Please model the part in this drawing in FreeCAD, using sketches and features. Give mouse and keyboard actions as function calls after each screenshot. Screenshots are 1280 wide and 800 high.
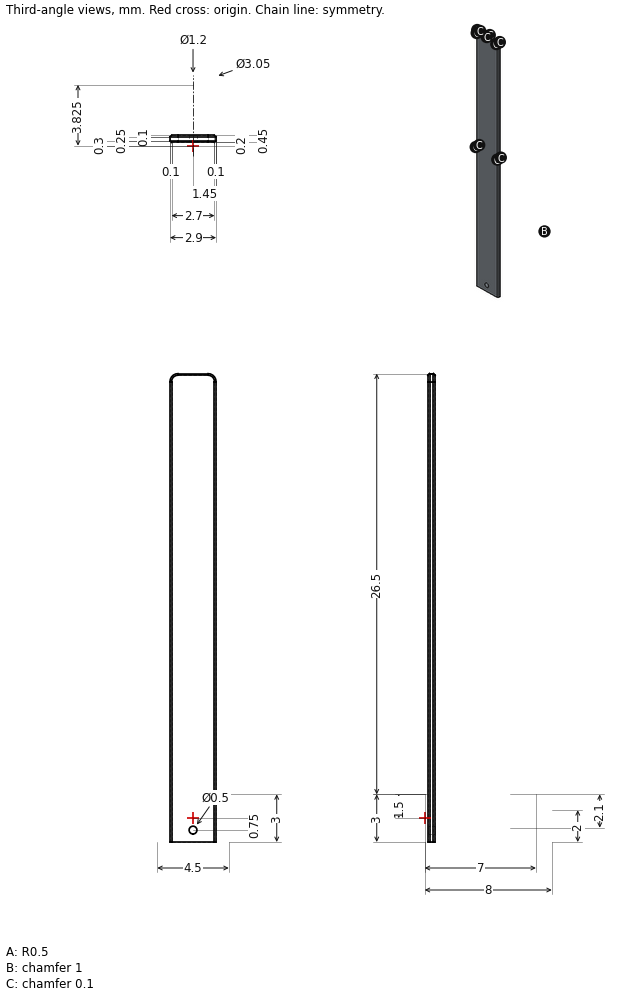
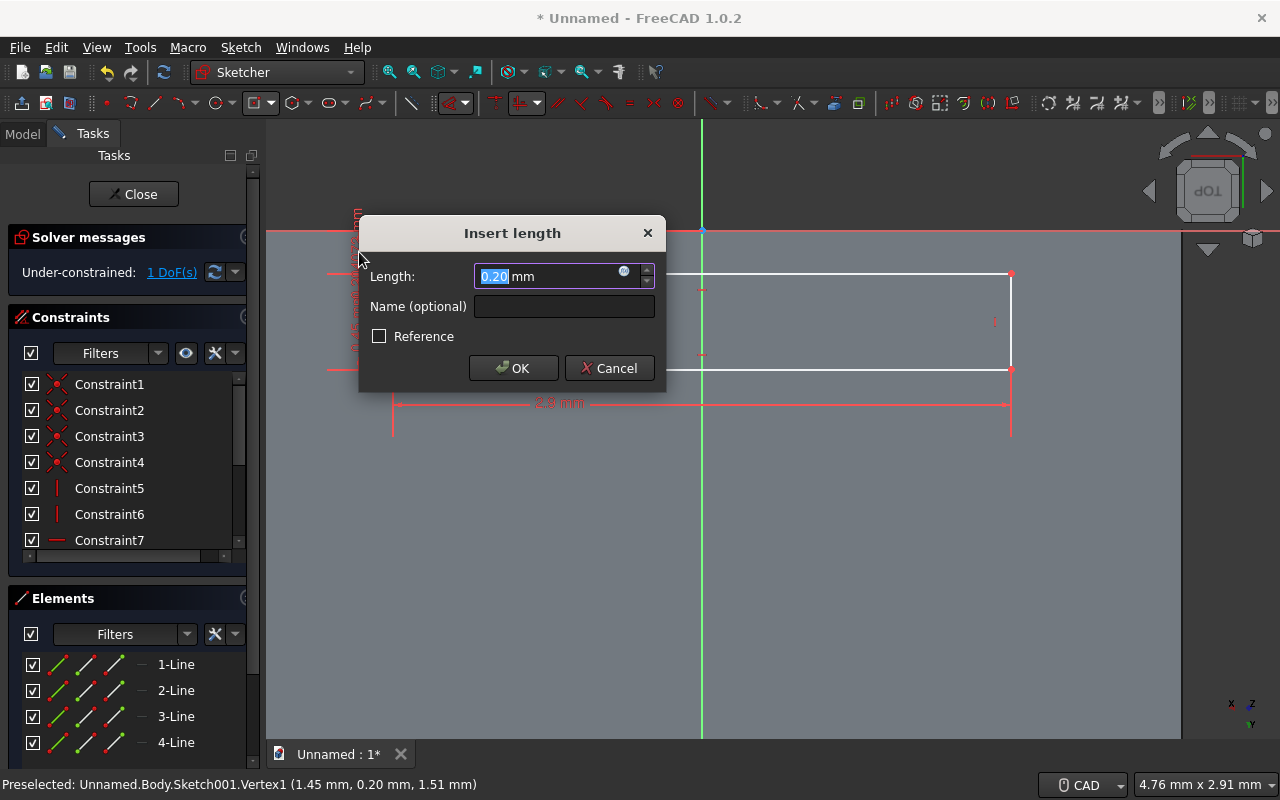
text(0.2)
key(Return)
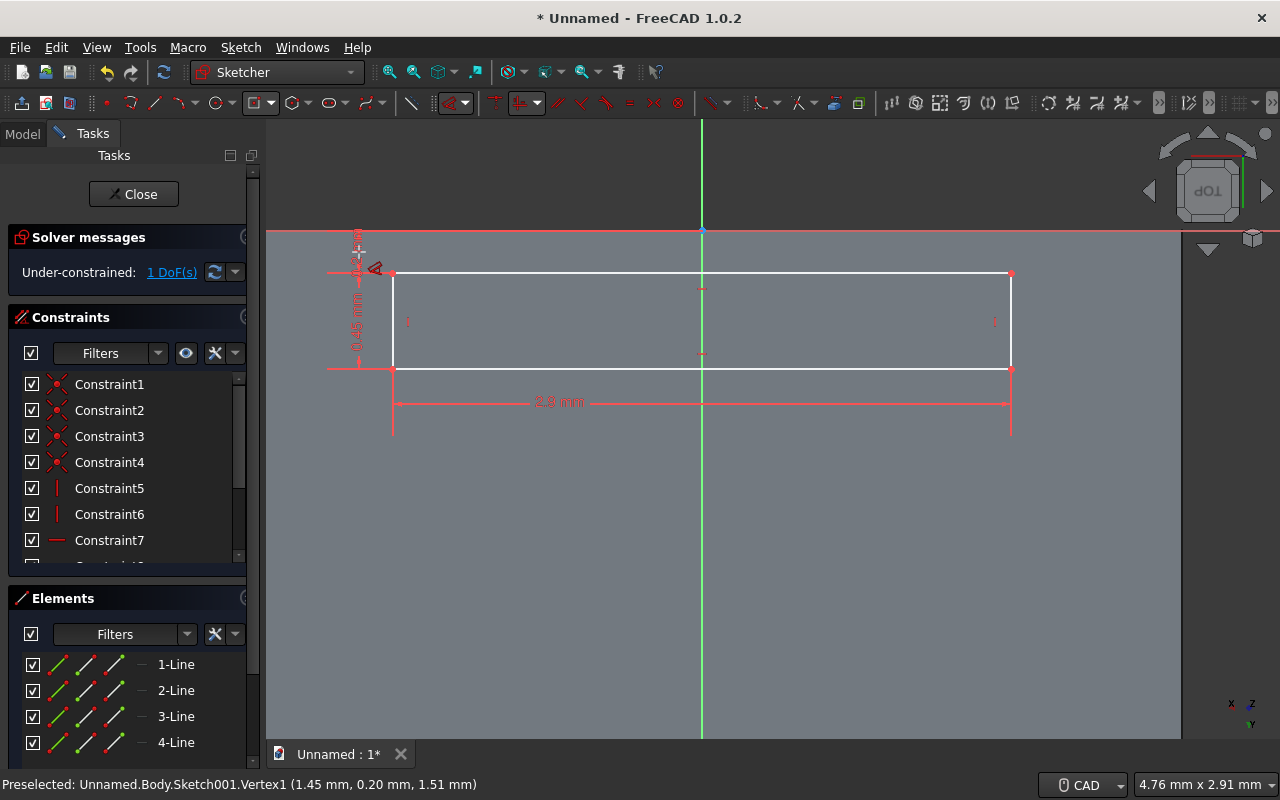
click(393, 273)
click(548, 196)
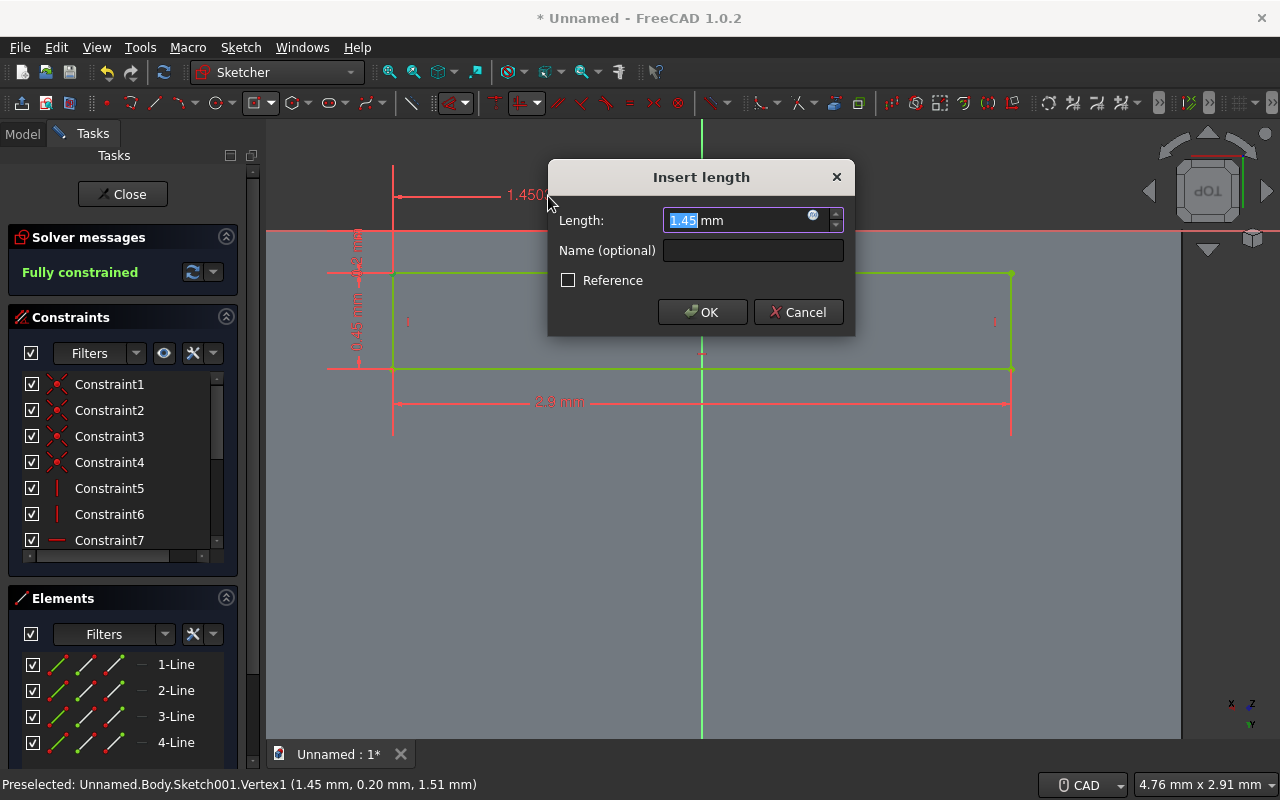
text(1.45)
key(Return)
key(Escape)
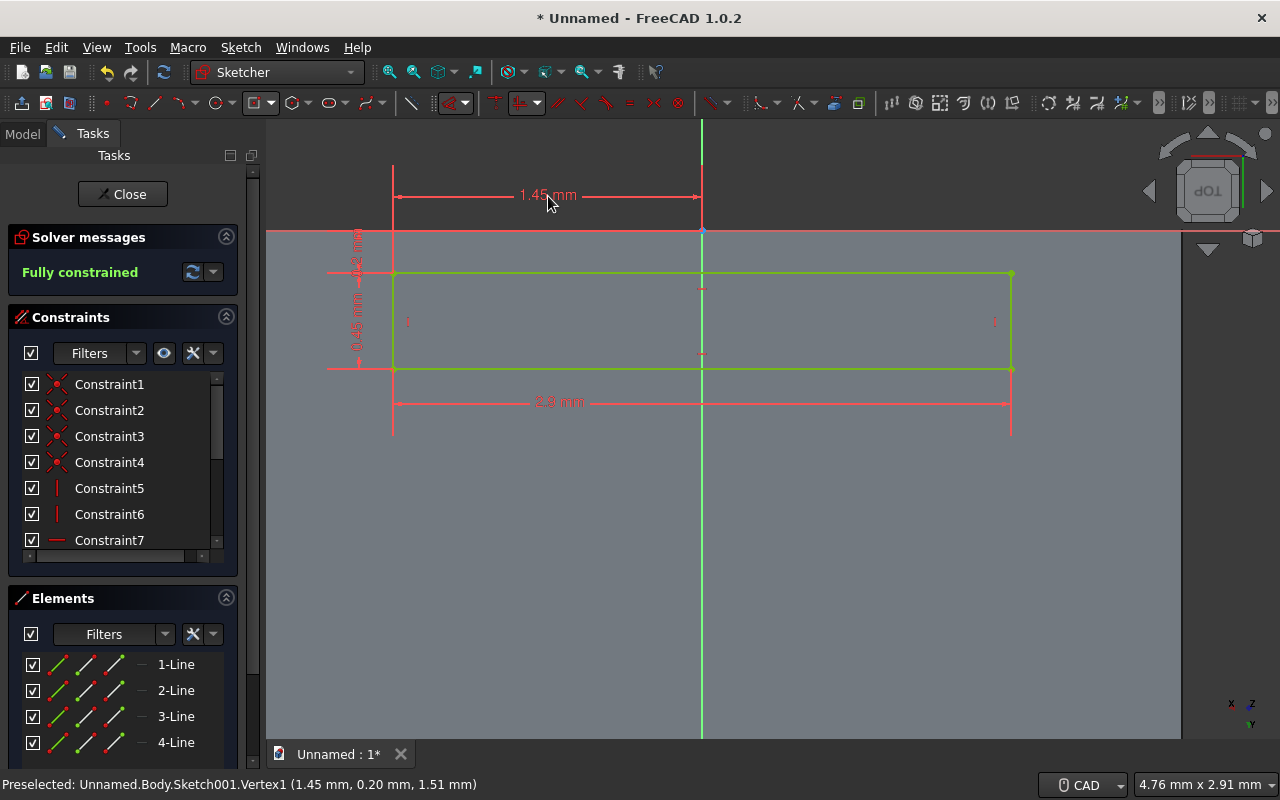
click(123, 194)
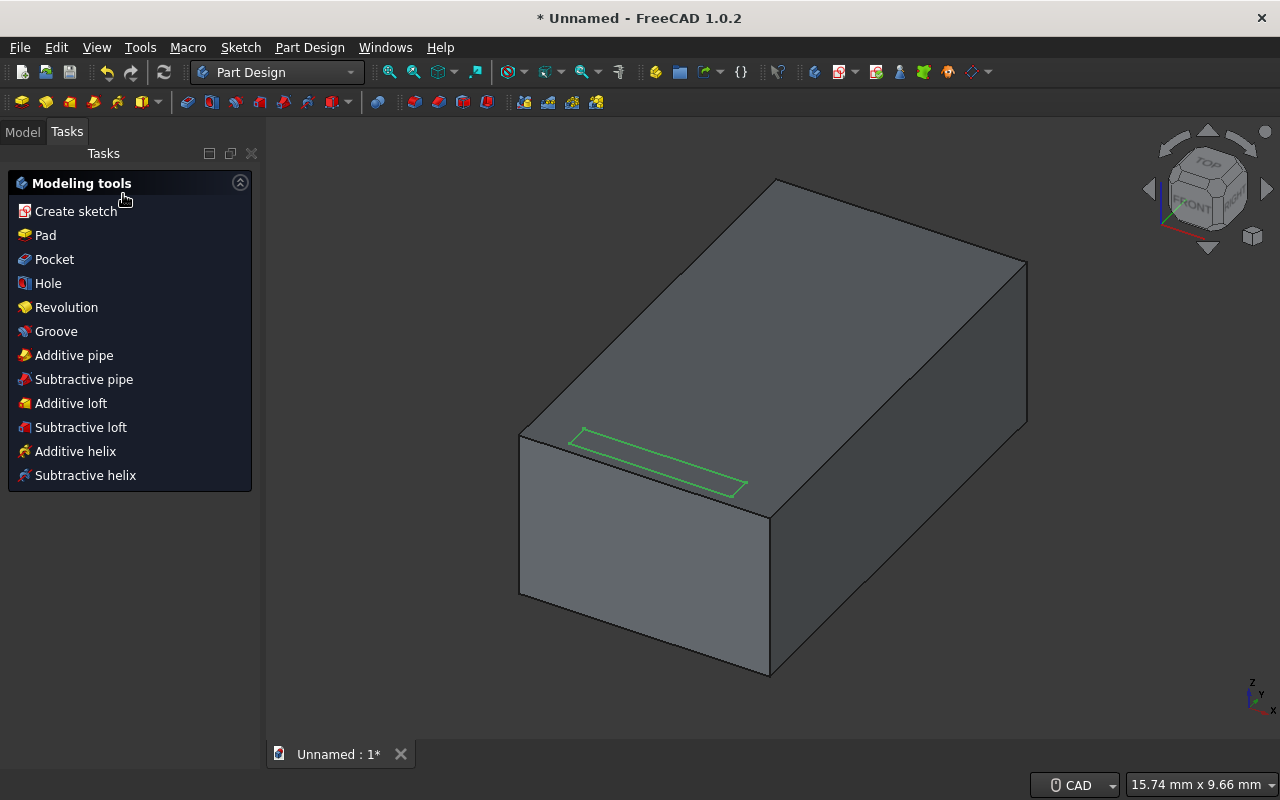
click(22, 102)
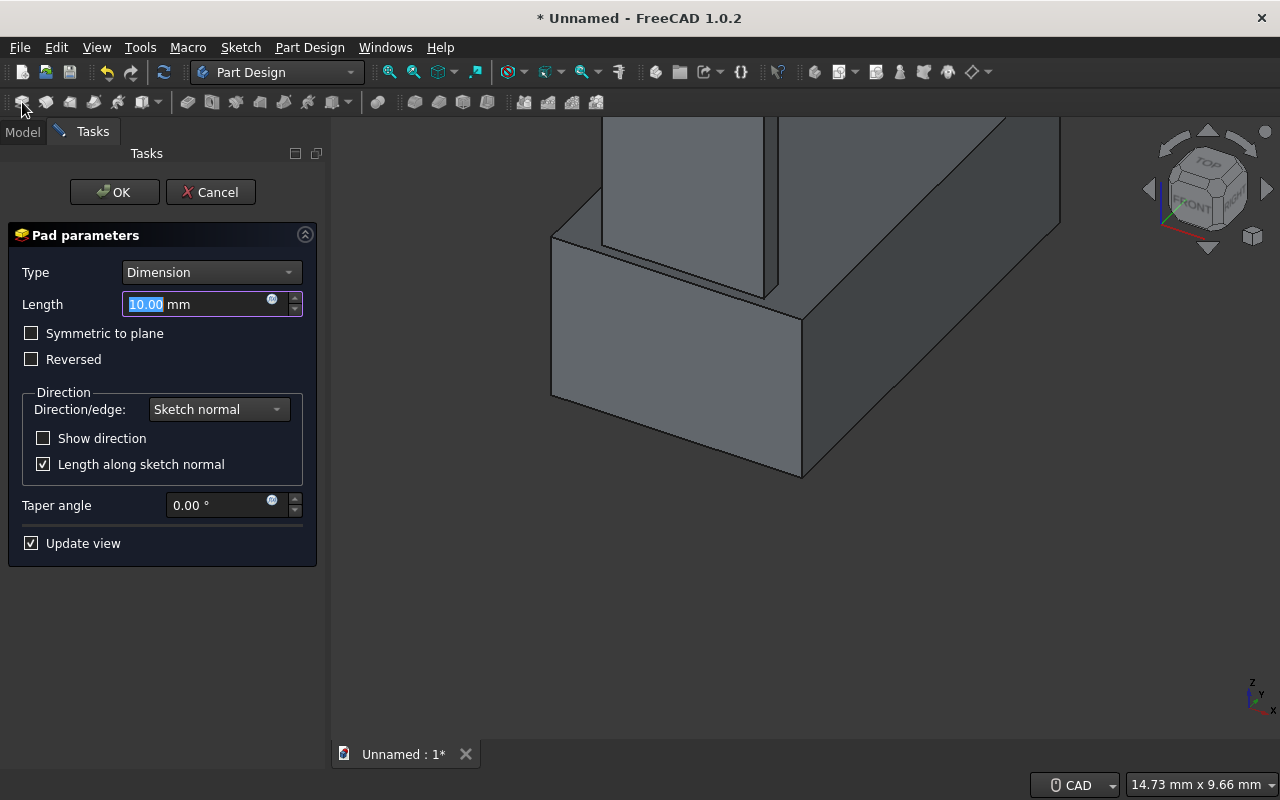
text(26.5)
key(Tab)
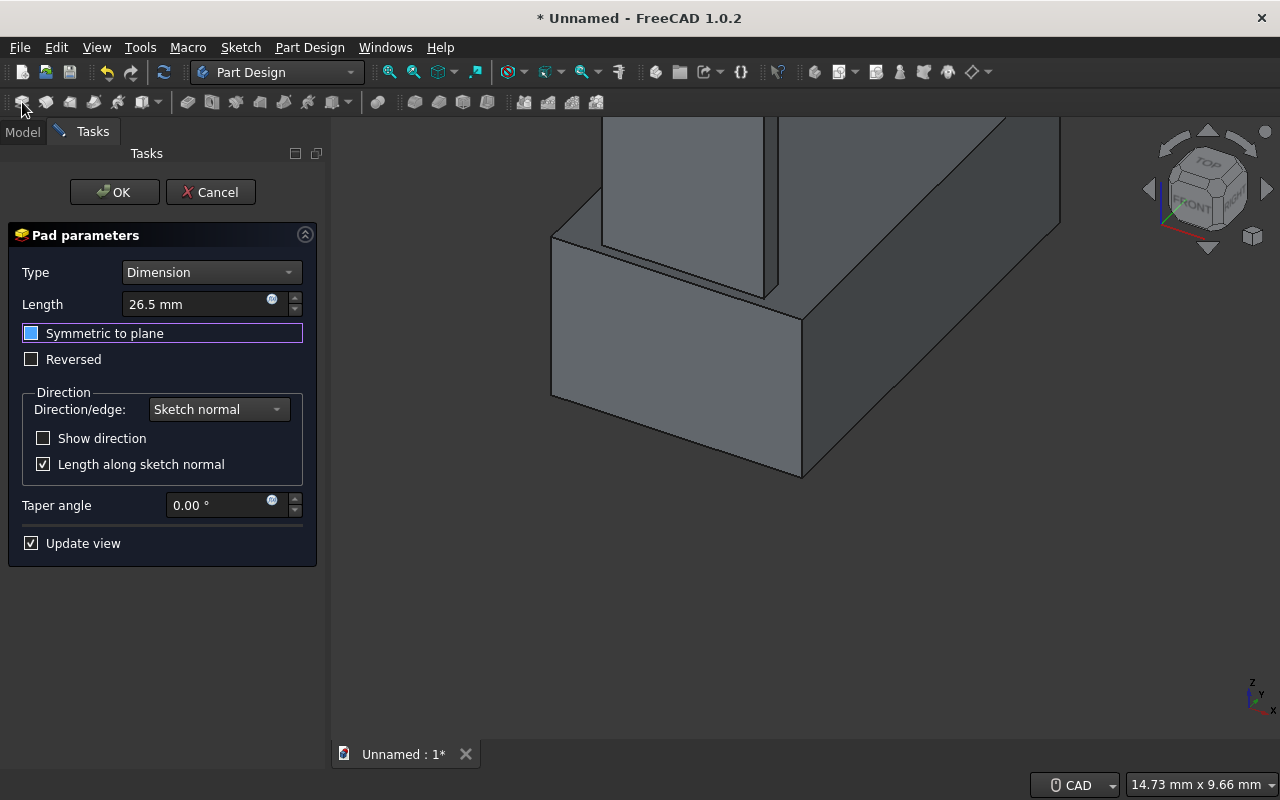
click(115, 192)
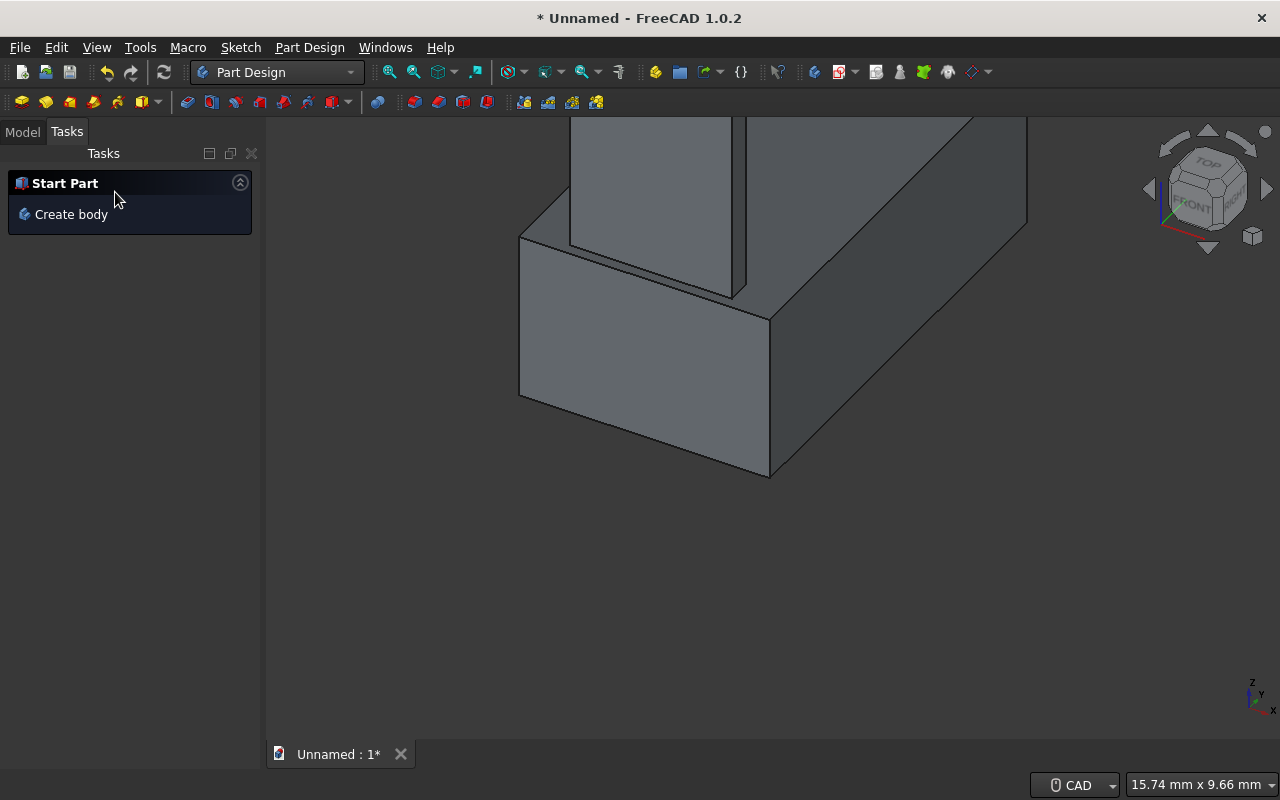
key(v)
key(f)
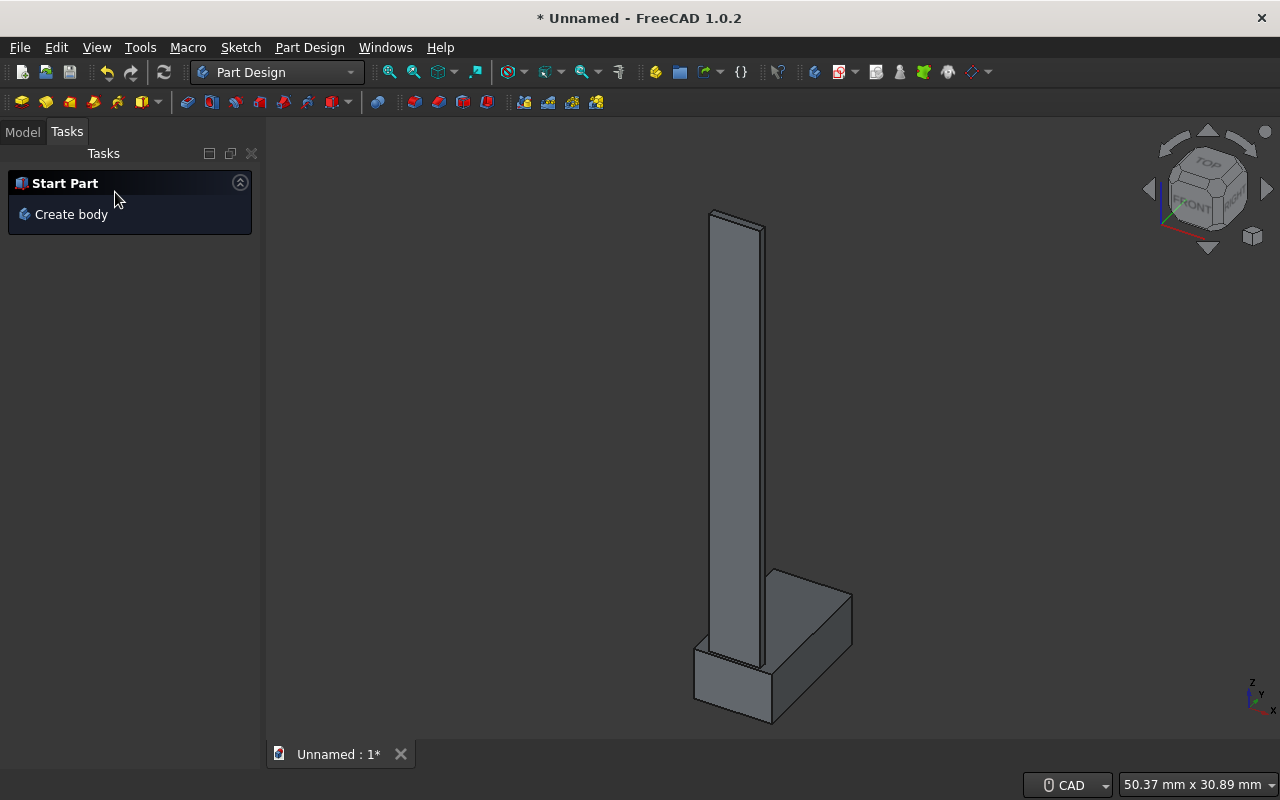
scroll(762, 228, up, 8)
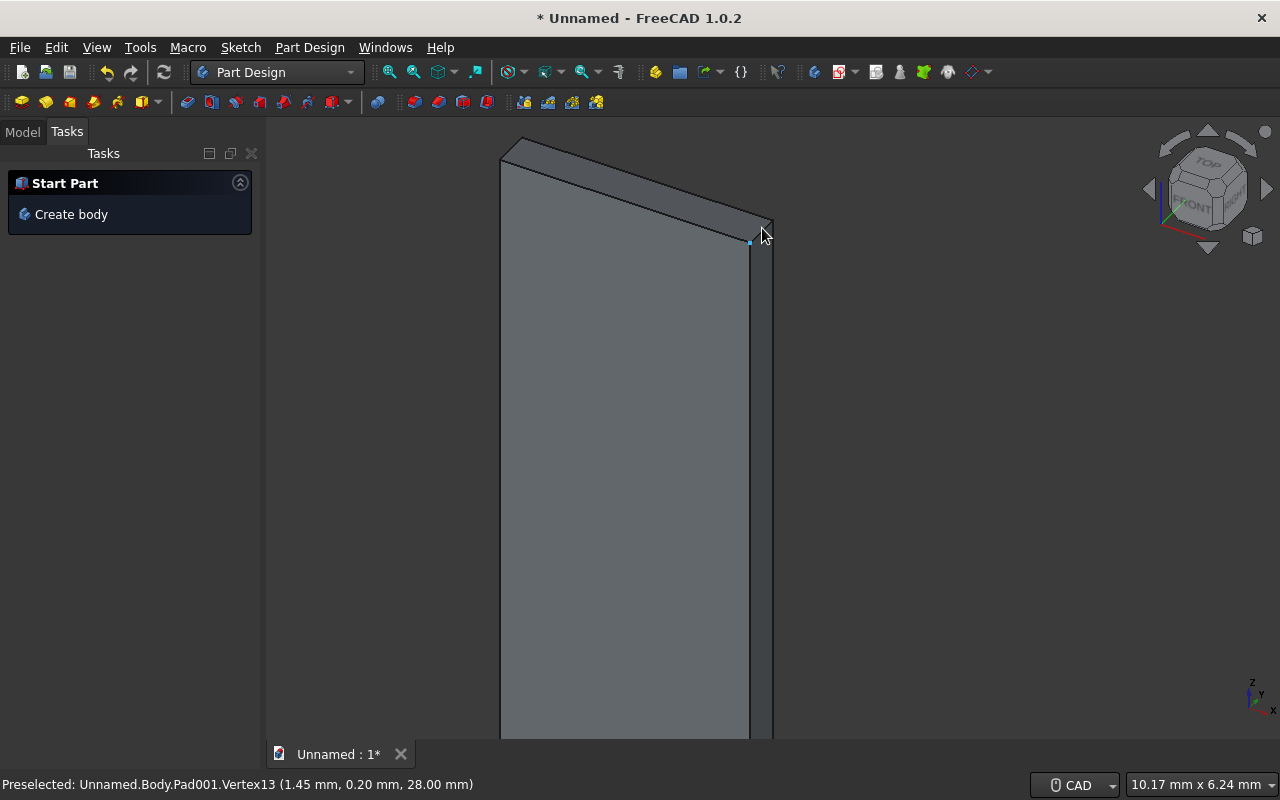
click(762, 231)